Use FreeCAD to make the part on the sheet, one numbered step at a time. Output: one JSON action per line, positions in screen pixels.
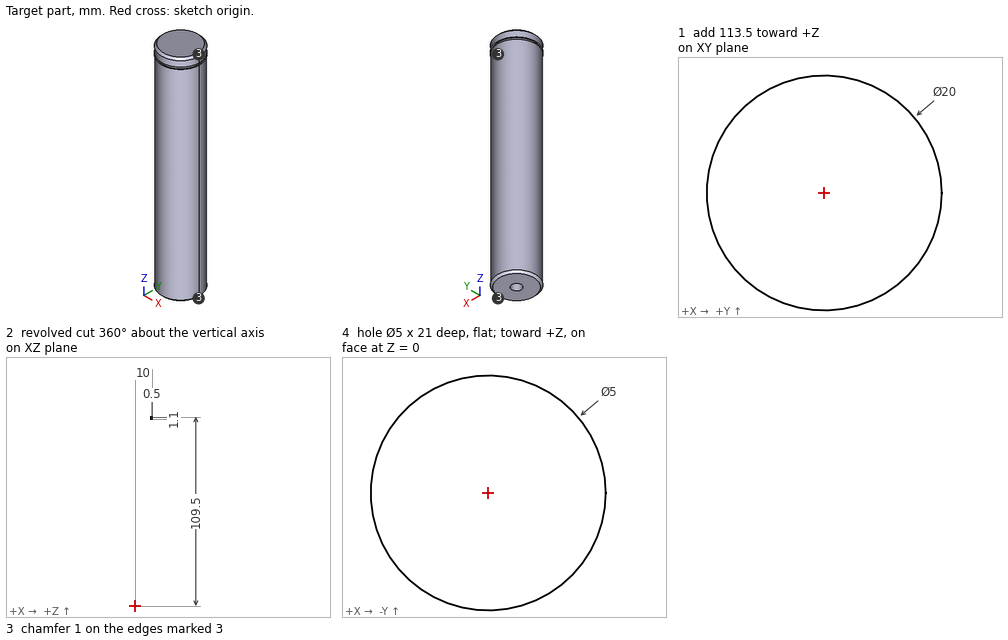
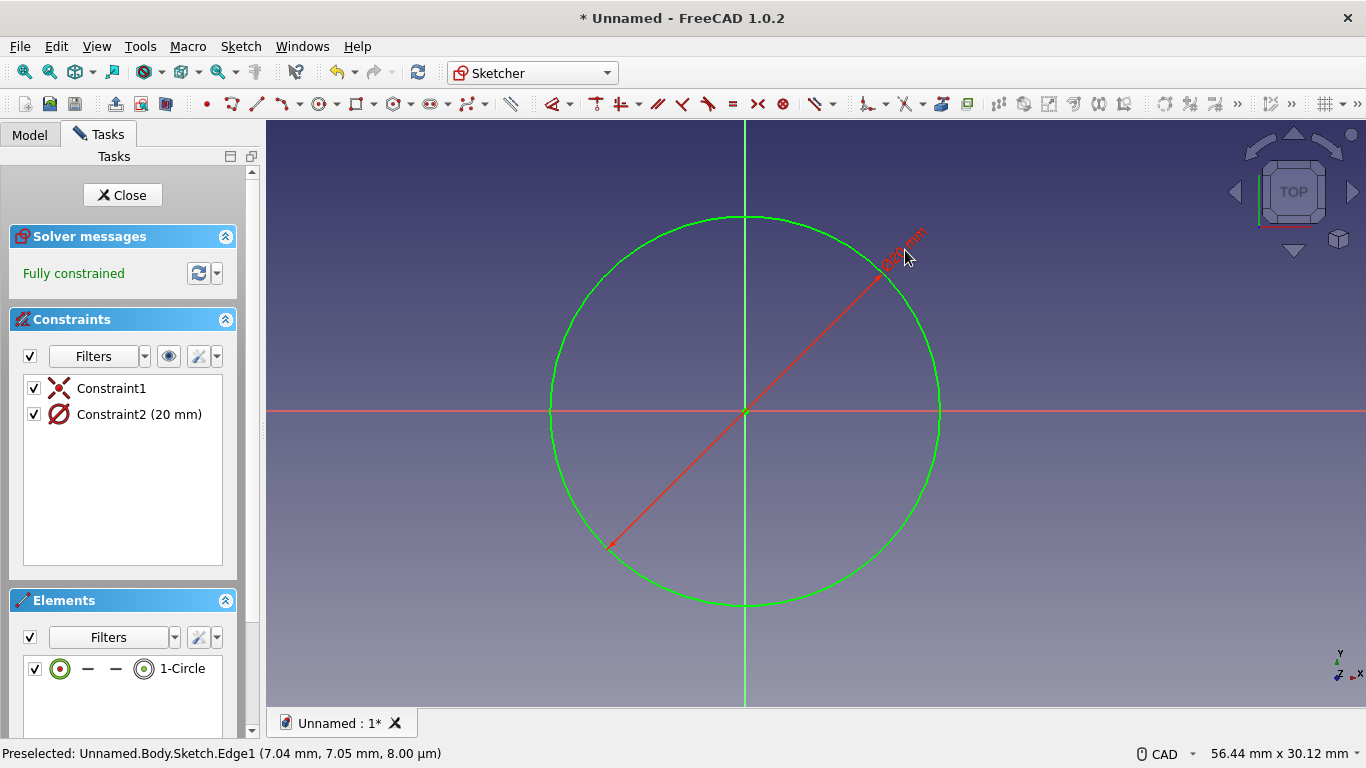
{"action": "left_click", "coordinate": [123, 195]}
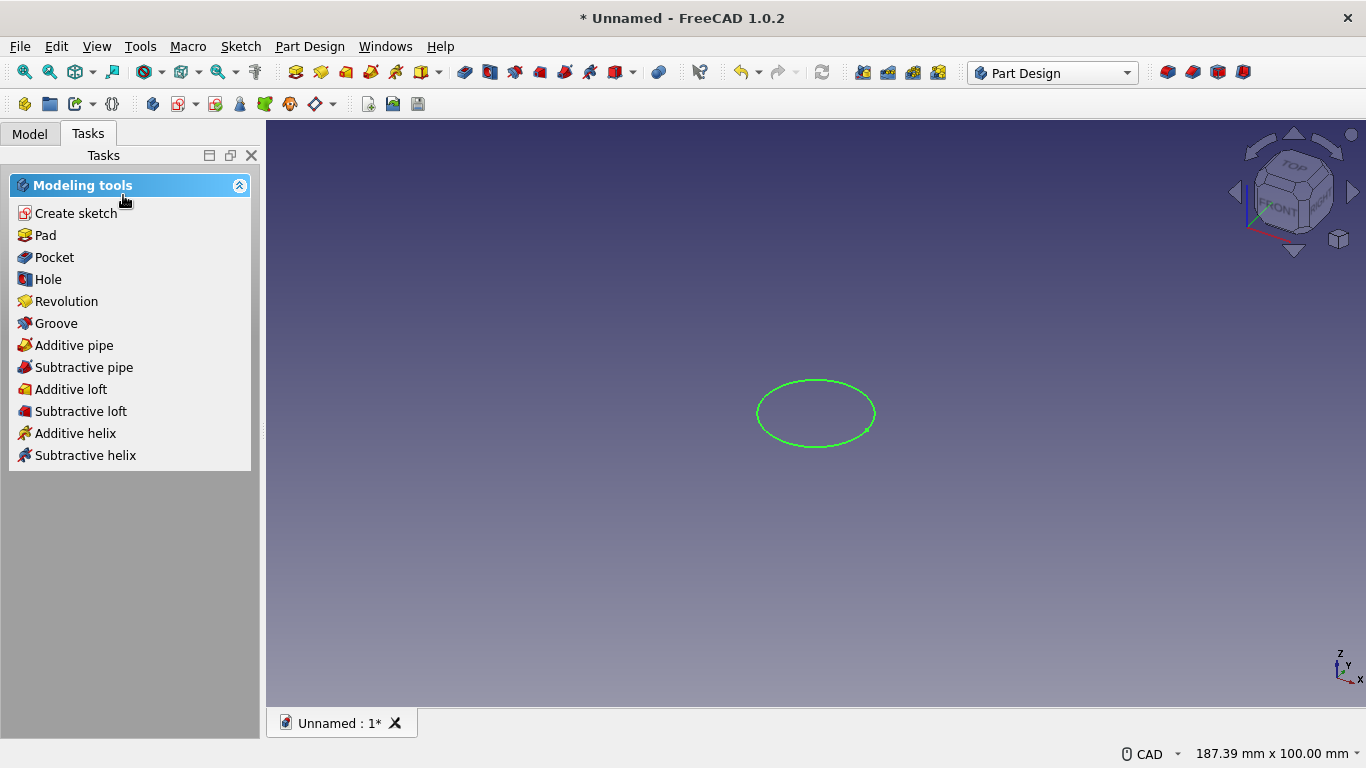
{"action": "left_click", "coordinate": [296, 72]}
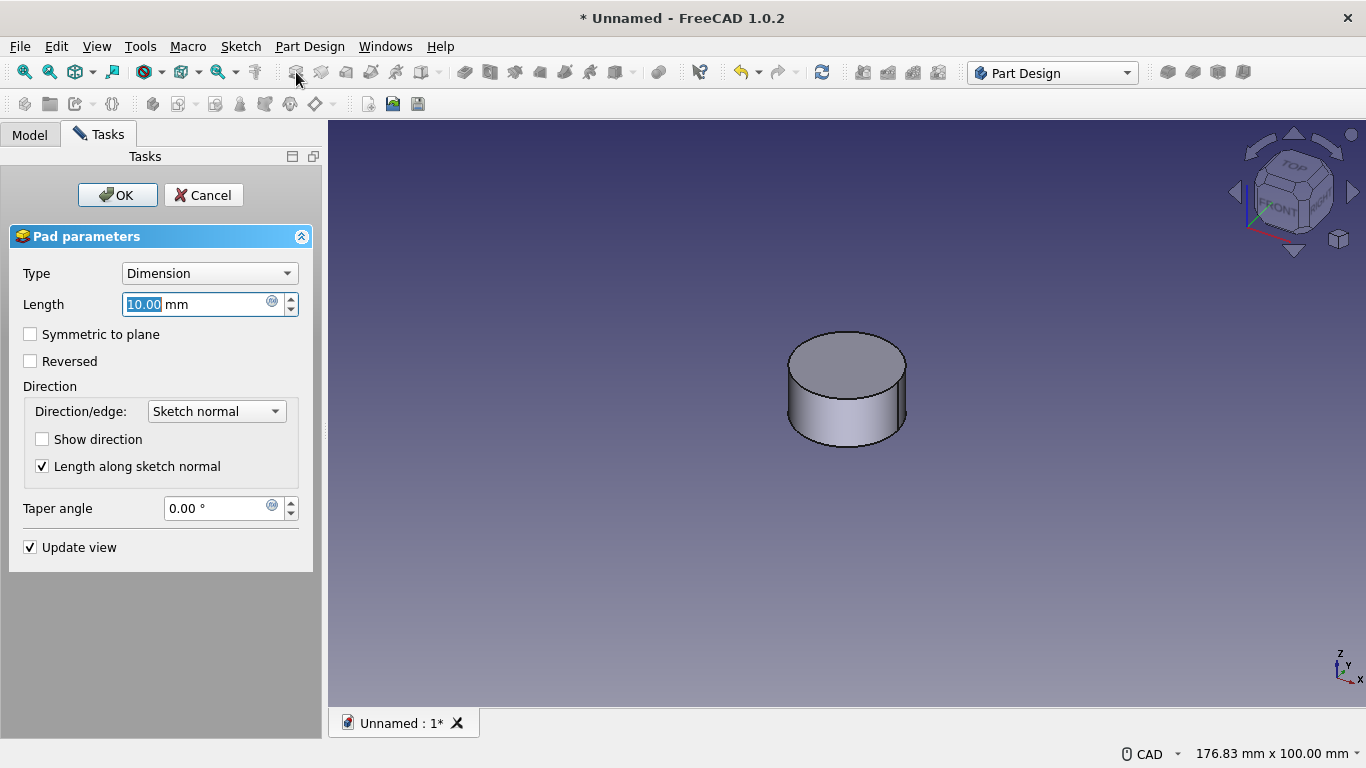
{"action": "type", "text": "113.5"}
{"action": "key", "text": "Tab"}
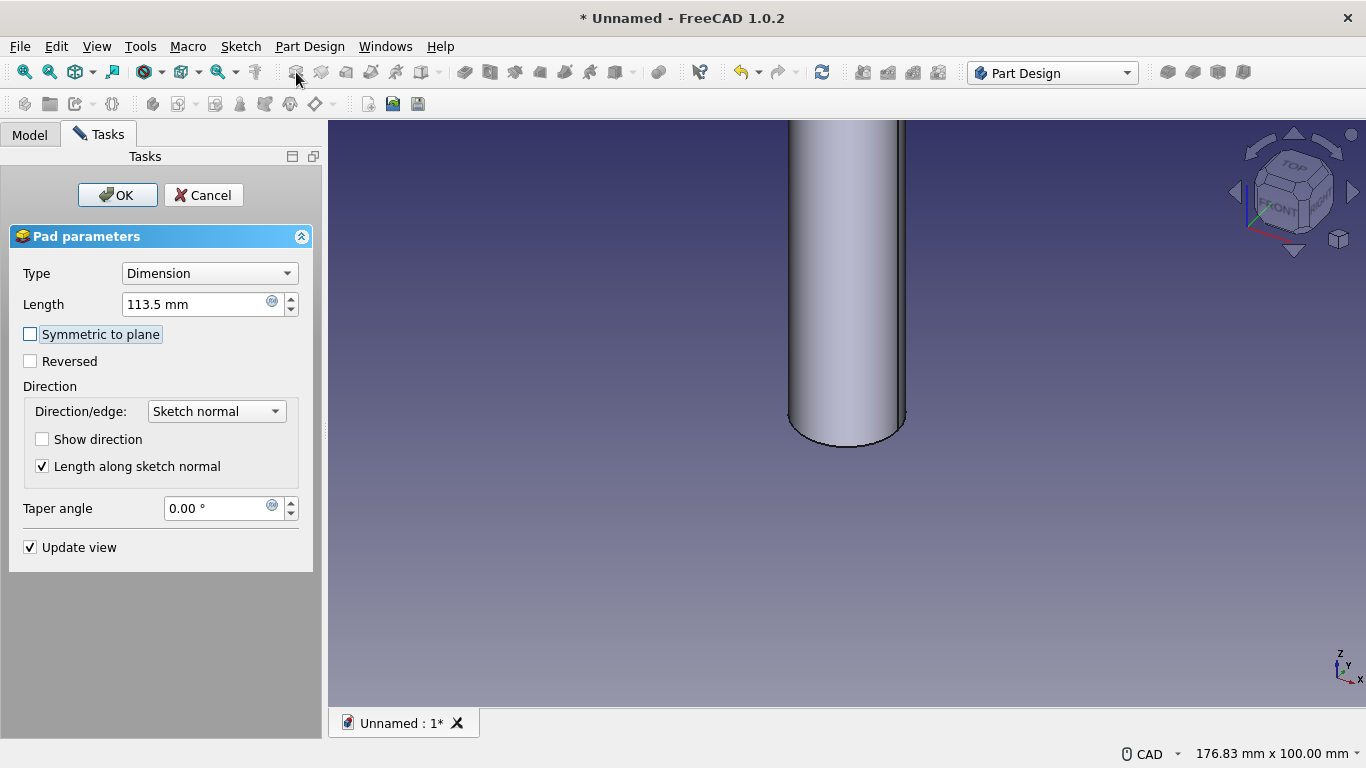
{"action": "left_click", "coordinate": [118, 195]}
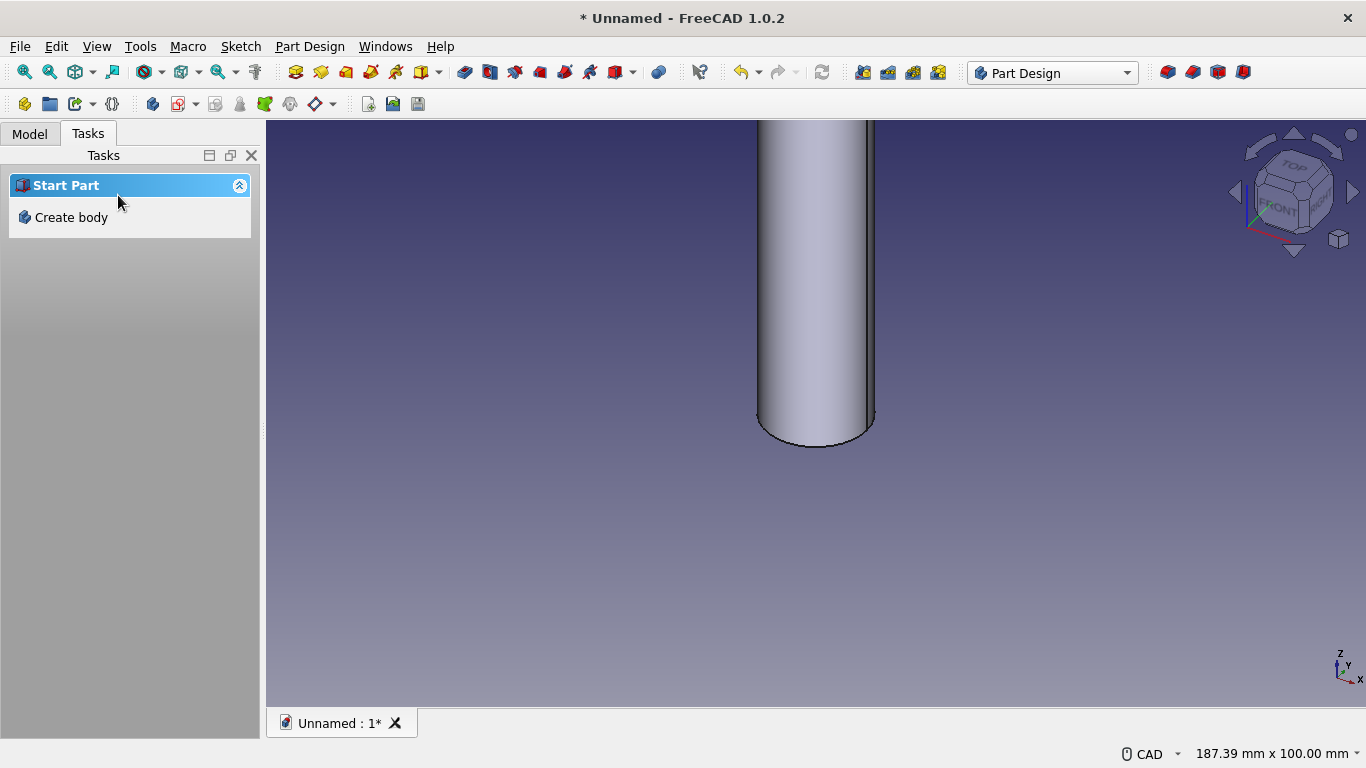
{"action": "key", "text": "v f"}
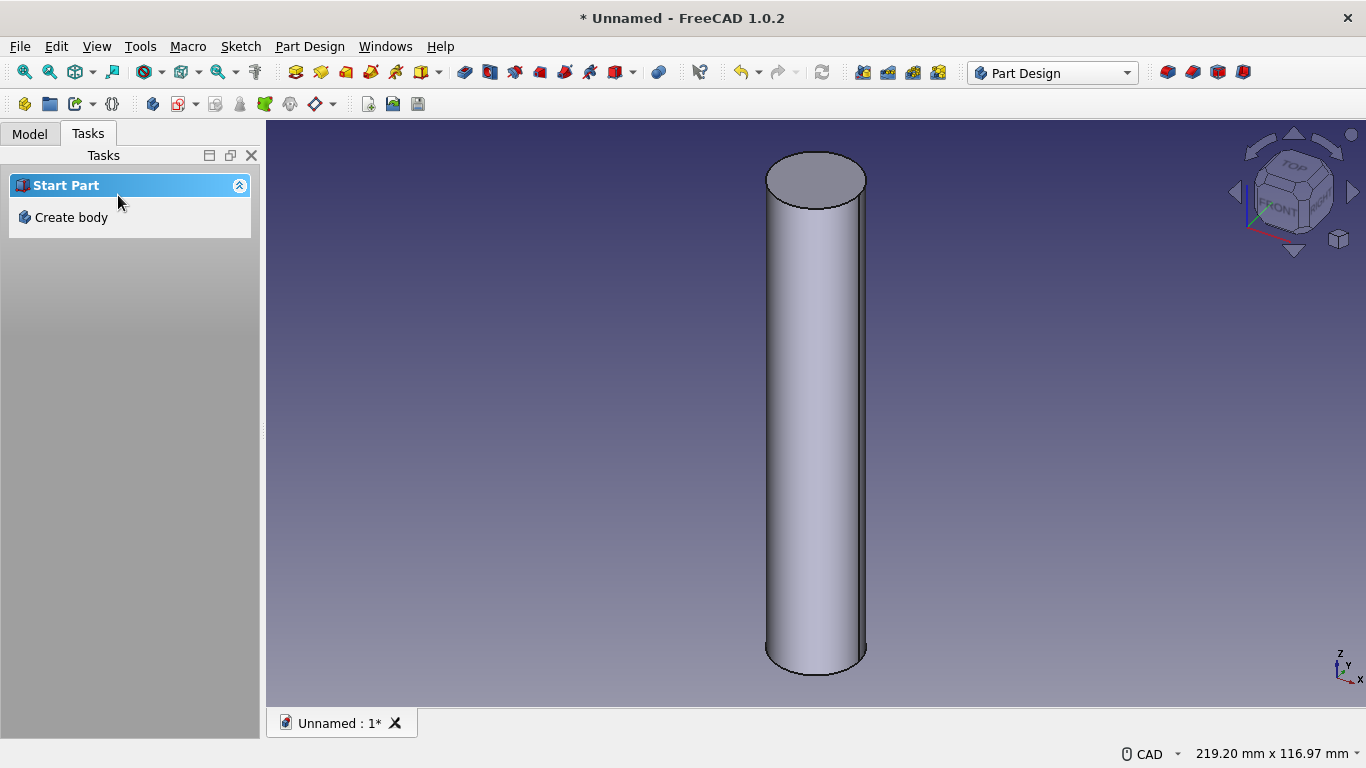
{"action": "left_click", "coordinate": [178, 104]}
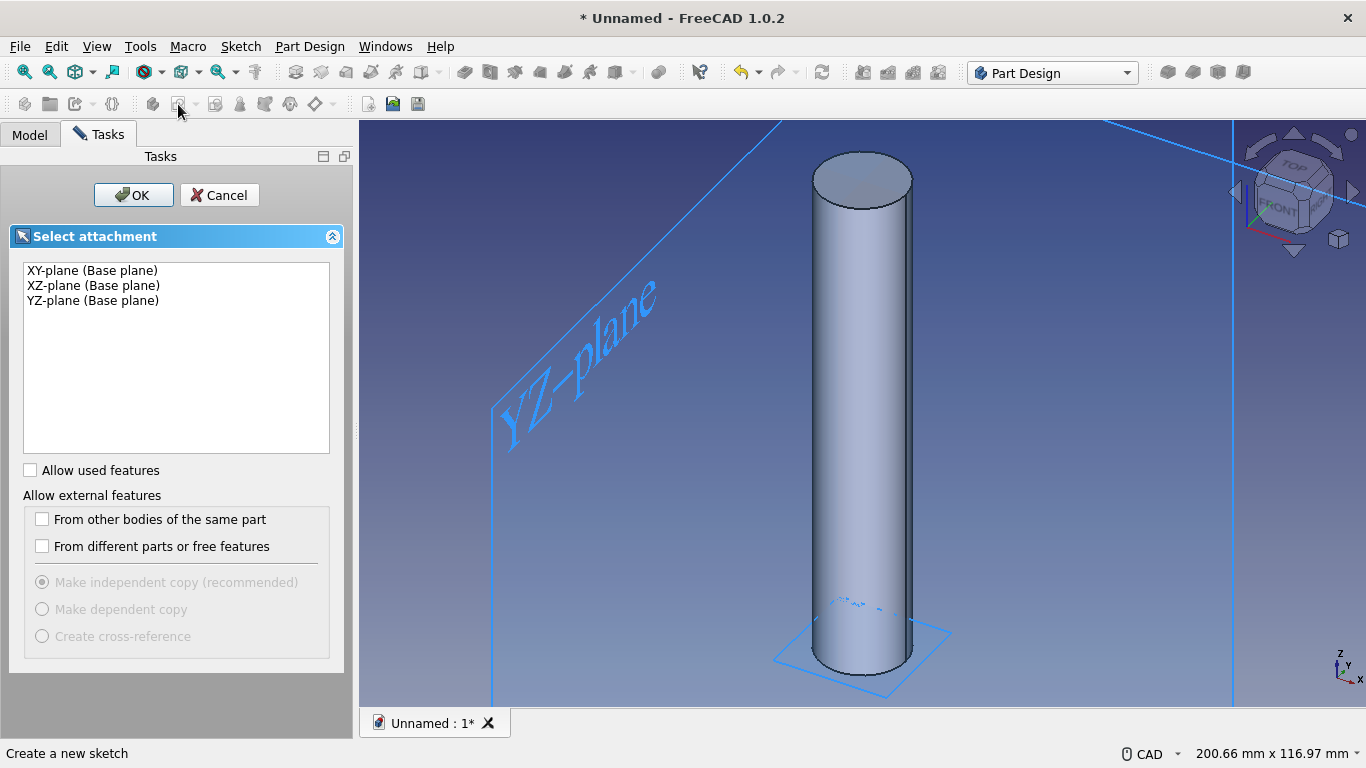
{"action": "left_click", "coordinate": [84, 286]}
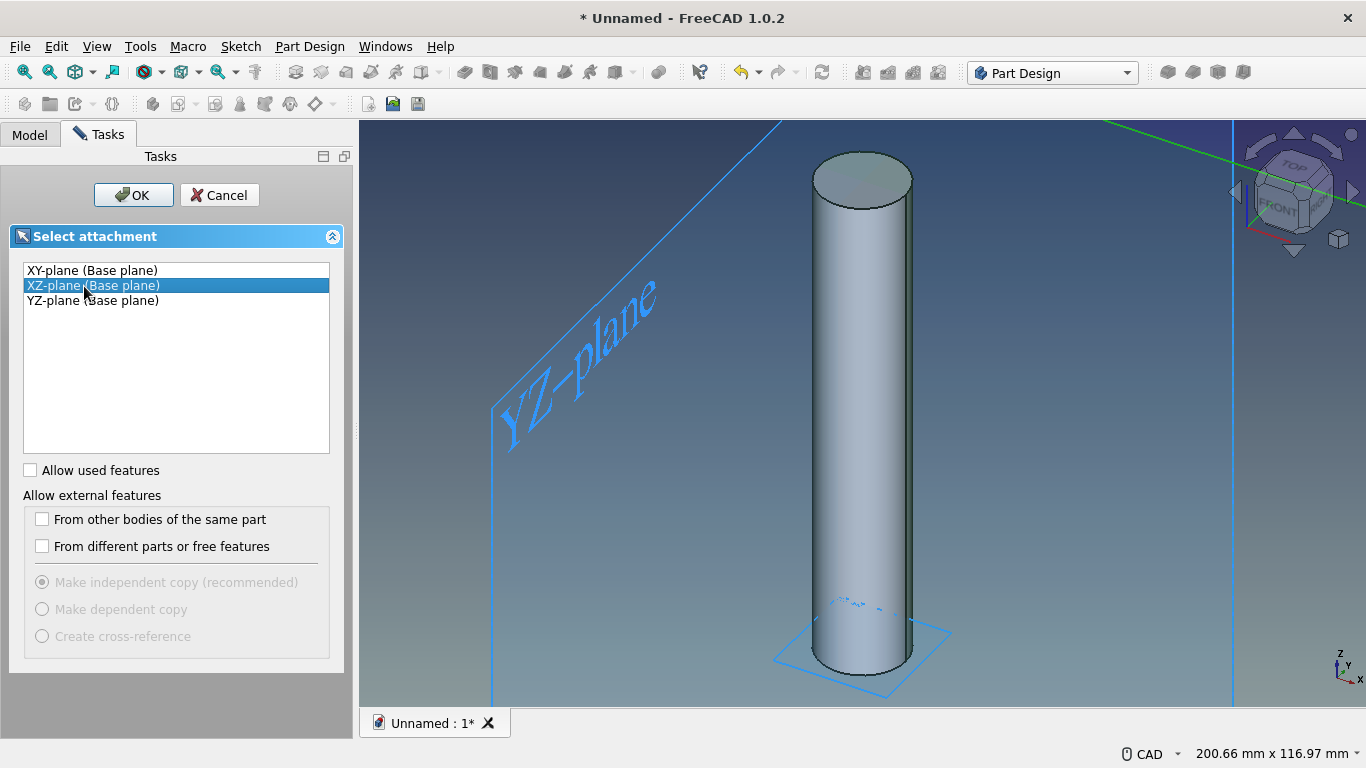
{"action": "left_click", "coordinate": [134, 195]}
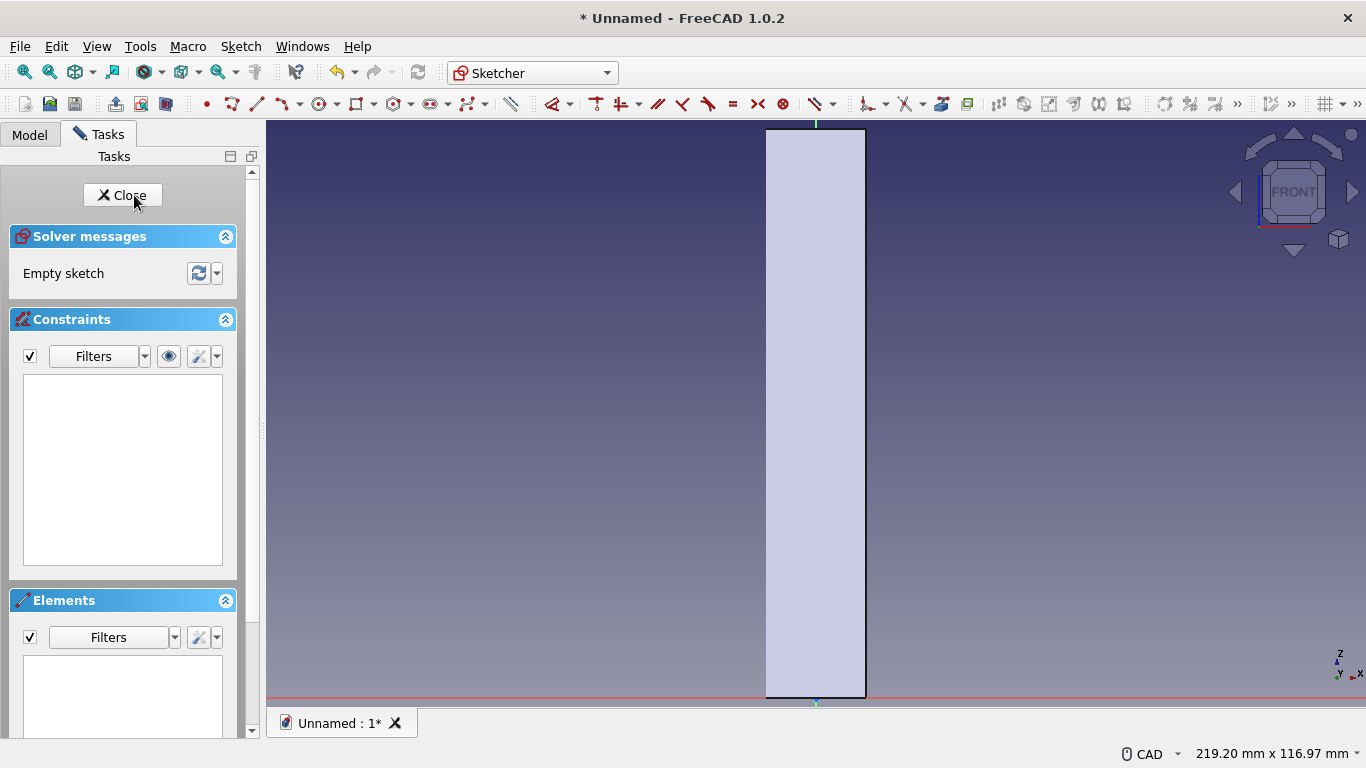
{"action": "key", "text": "q s"}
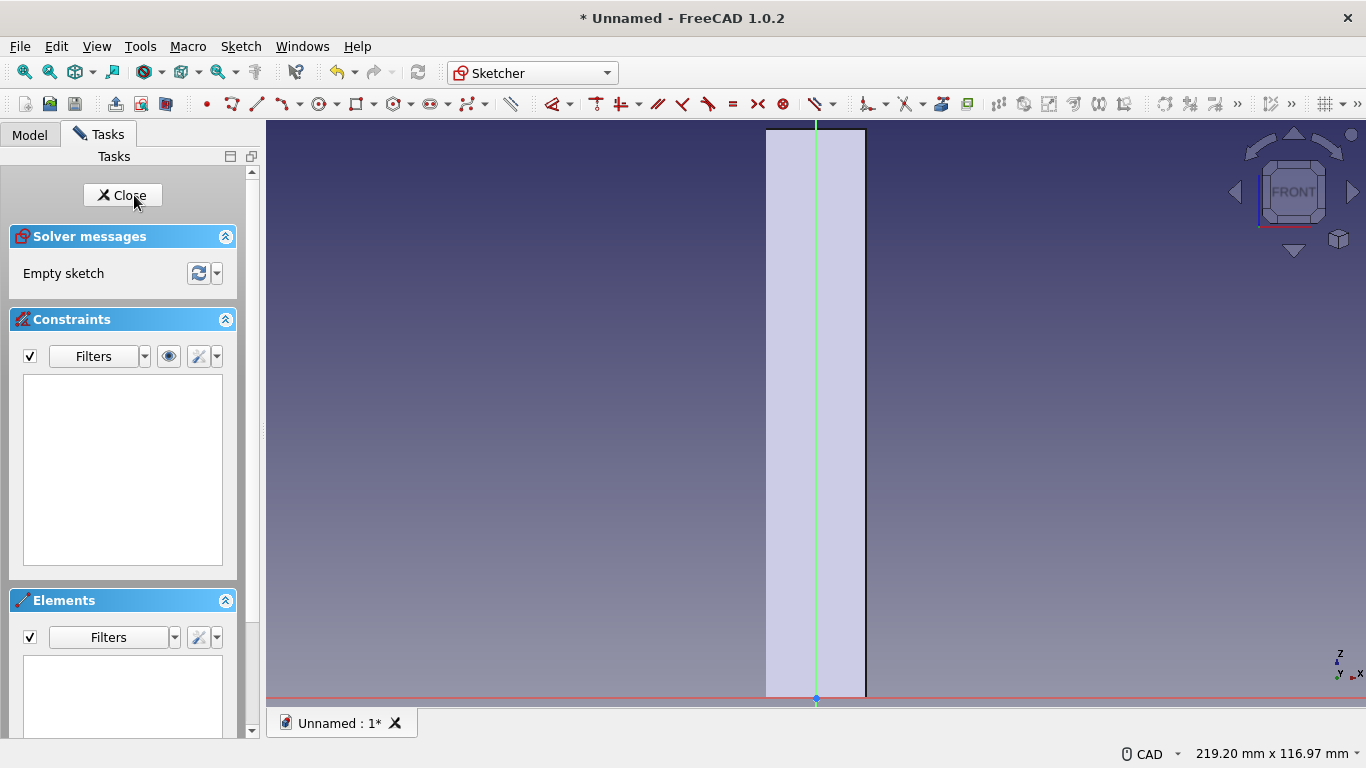
{"action": "scroll", "coordinate": [748, 414], "scroll_direction": "down", "scroll_amount": 5}